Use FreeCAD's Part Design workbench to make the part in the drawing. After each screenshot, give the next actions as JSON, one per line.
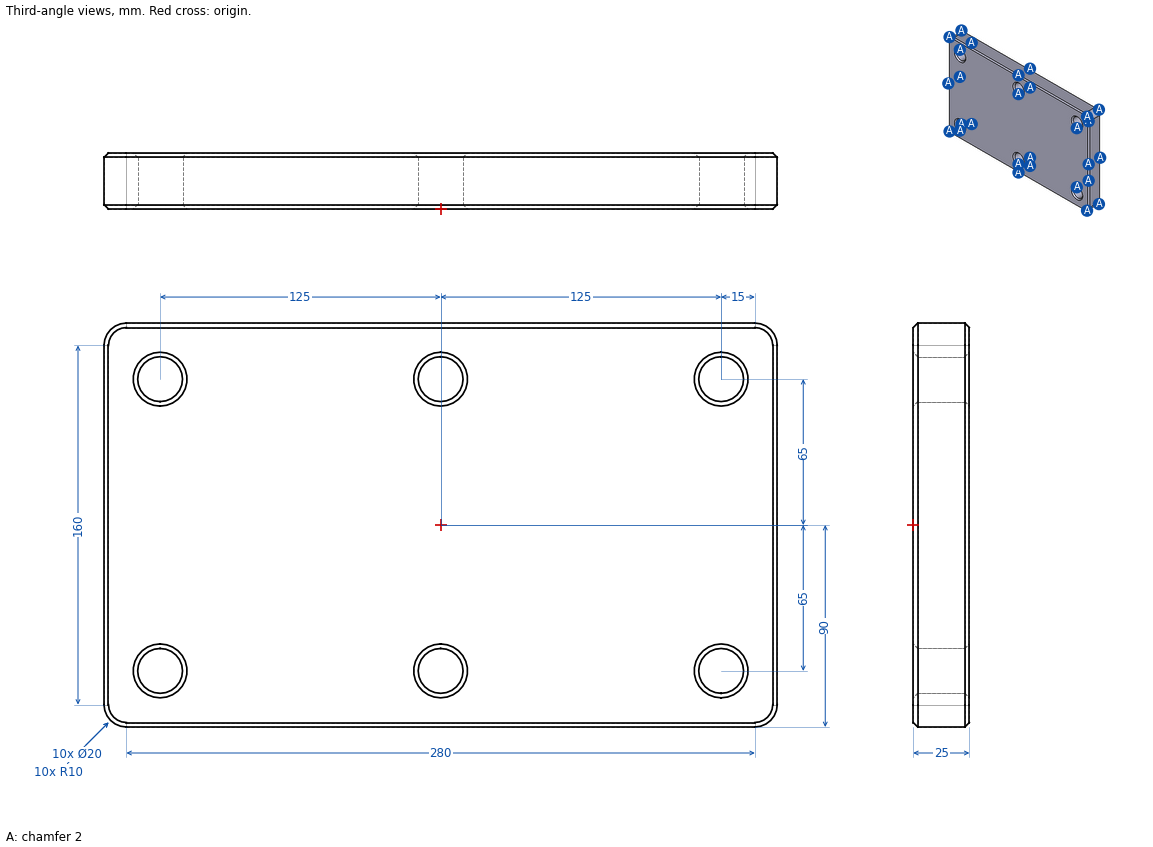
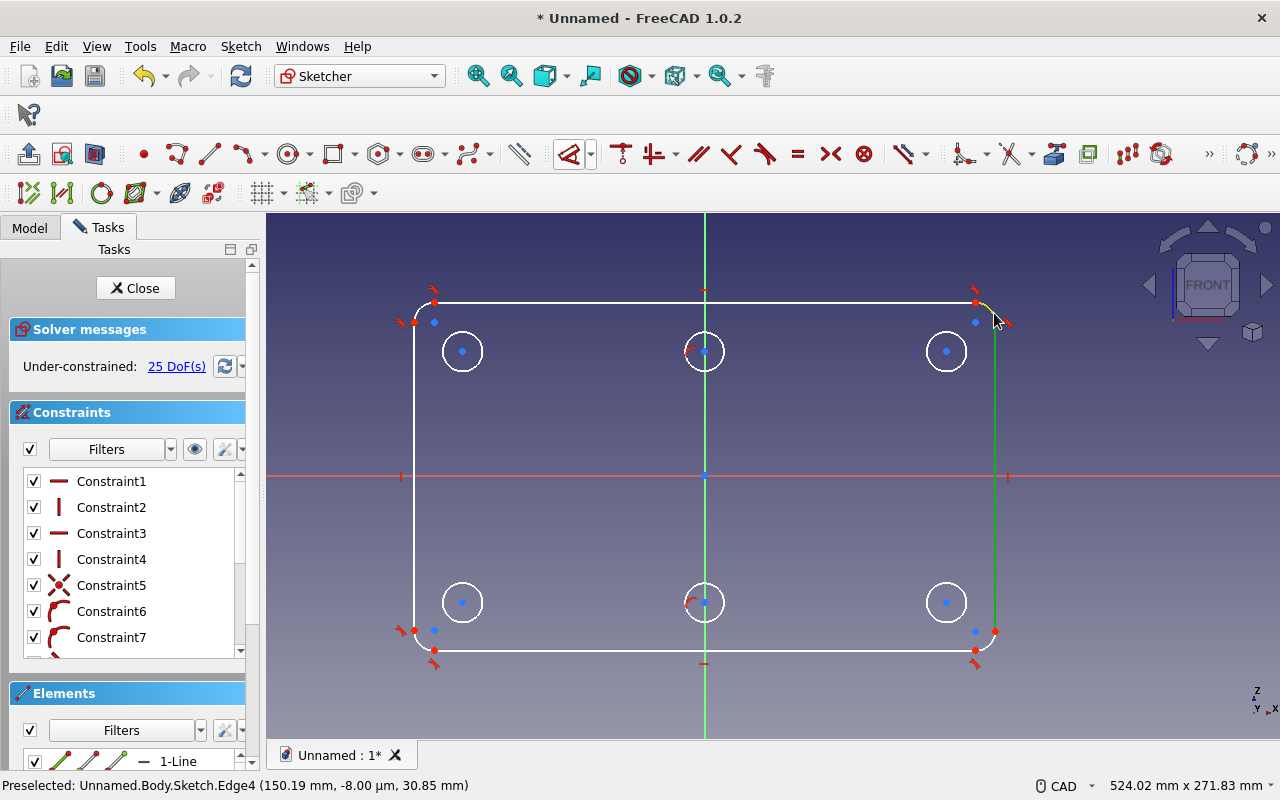
{"action": "scroll", "coordinate": [984, 649], "scroll_direction": "up", "scroll_amount": 3}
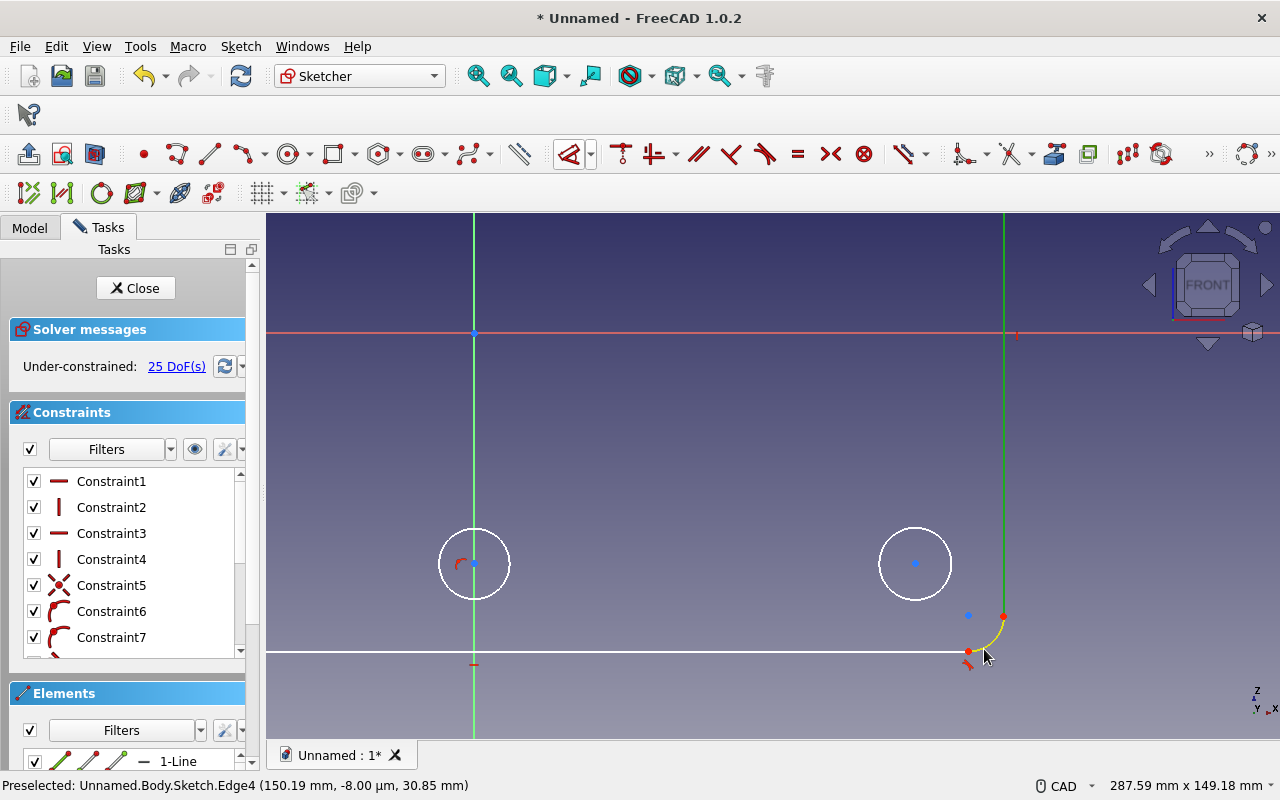
{"action": "left_click", "coordinate": [984, 648]}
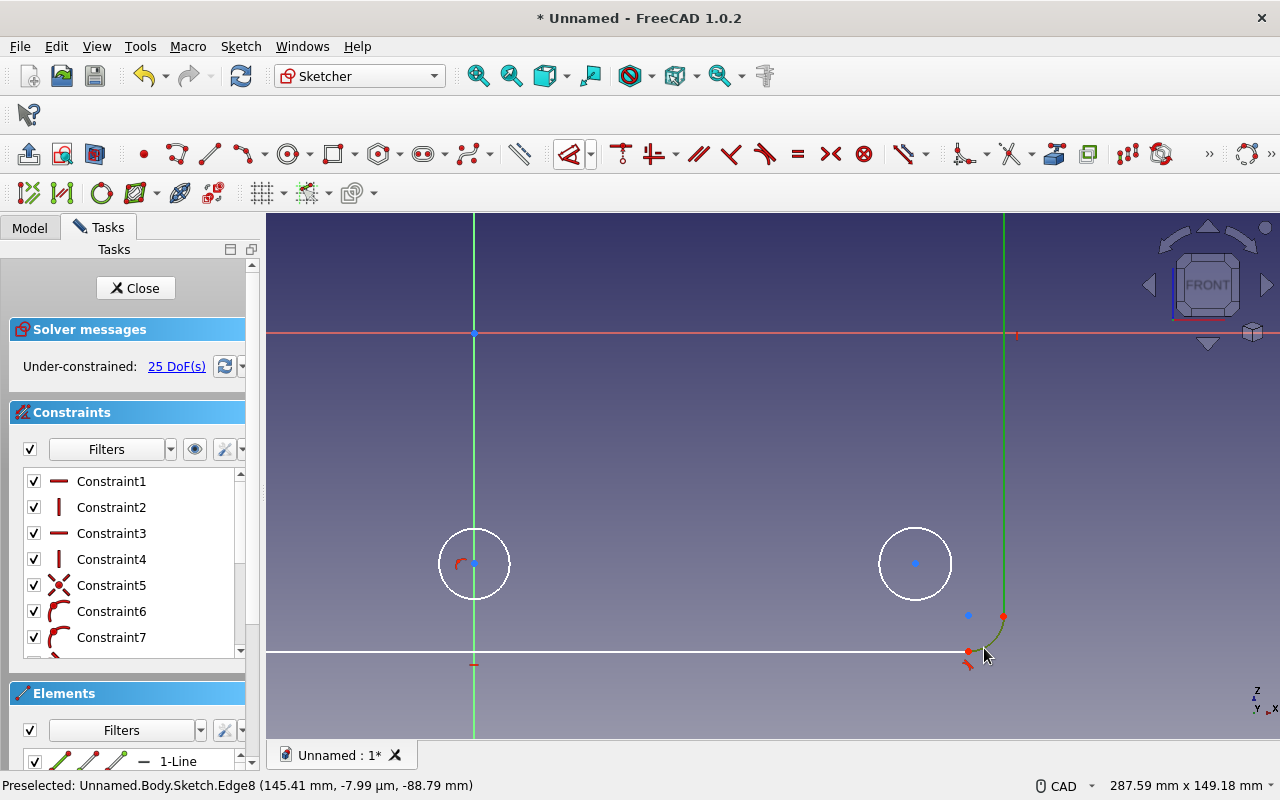
{"action": "left_click", "coordinate": [765, 154]}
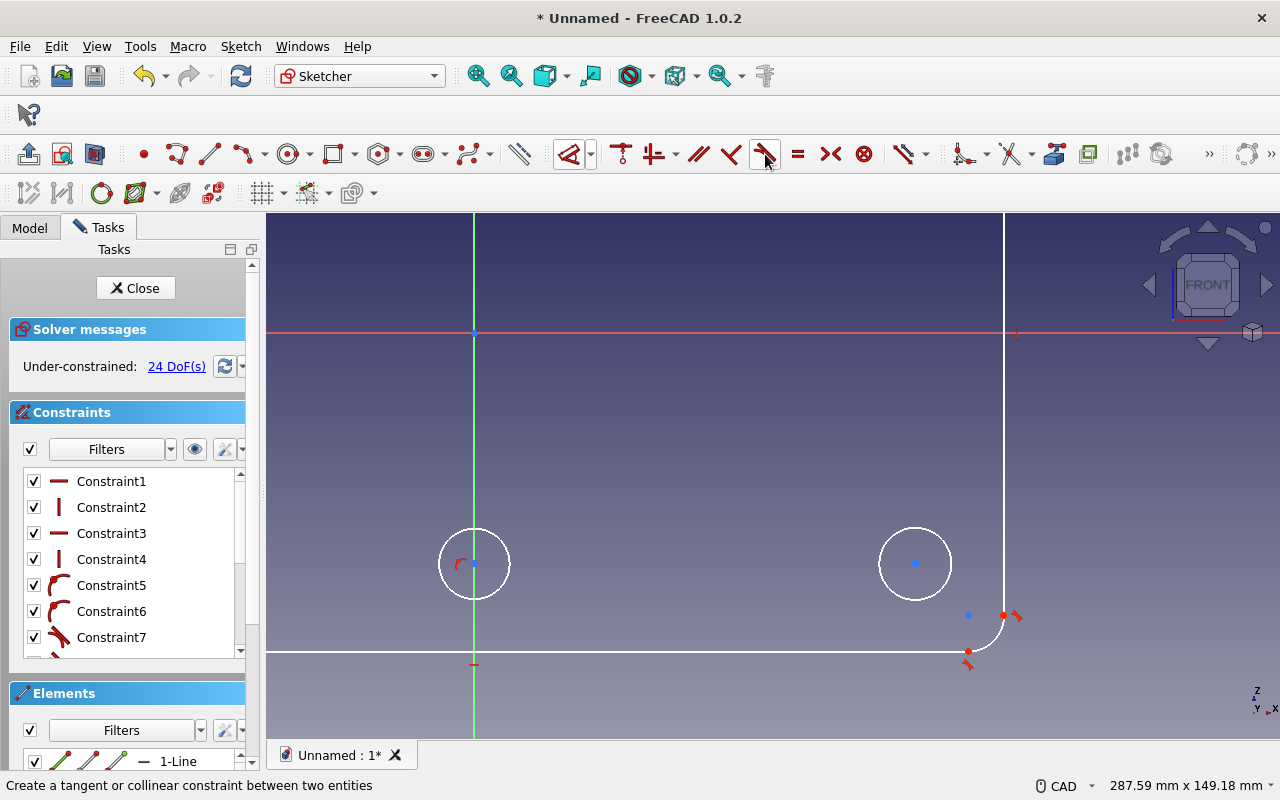
{"action": "scroll", "coordinate": [984, 650], "scroll_direction": "down", "scroll_amount": 3}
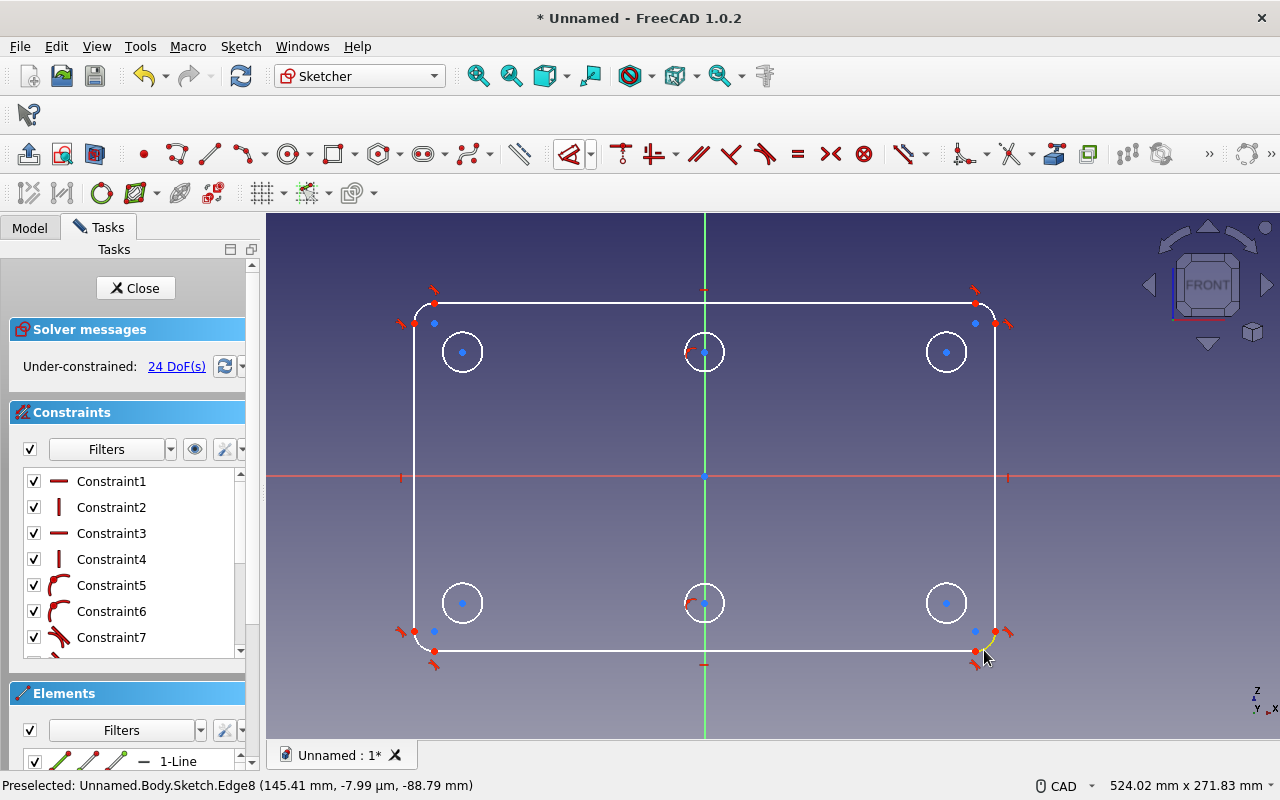
{"action": "scroll", "coordinate": [416, 640], "scroll_direction": "up", "scroll_amount": 3}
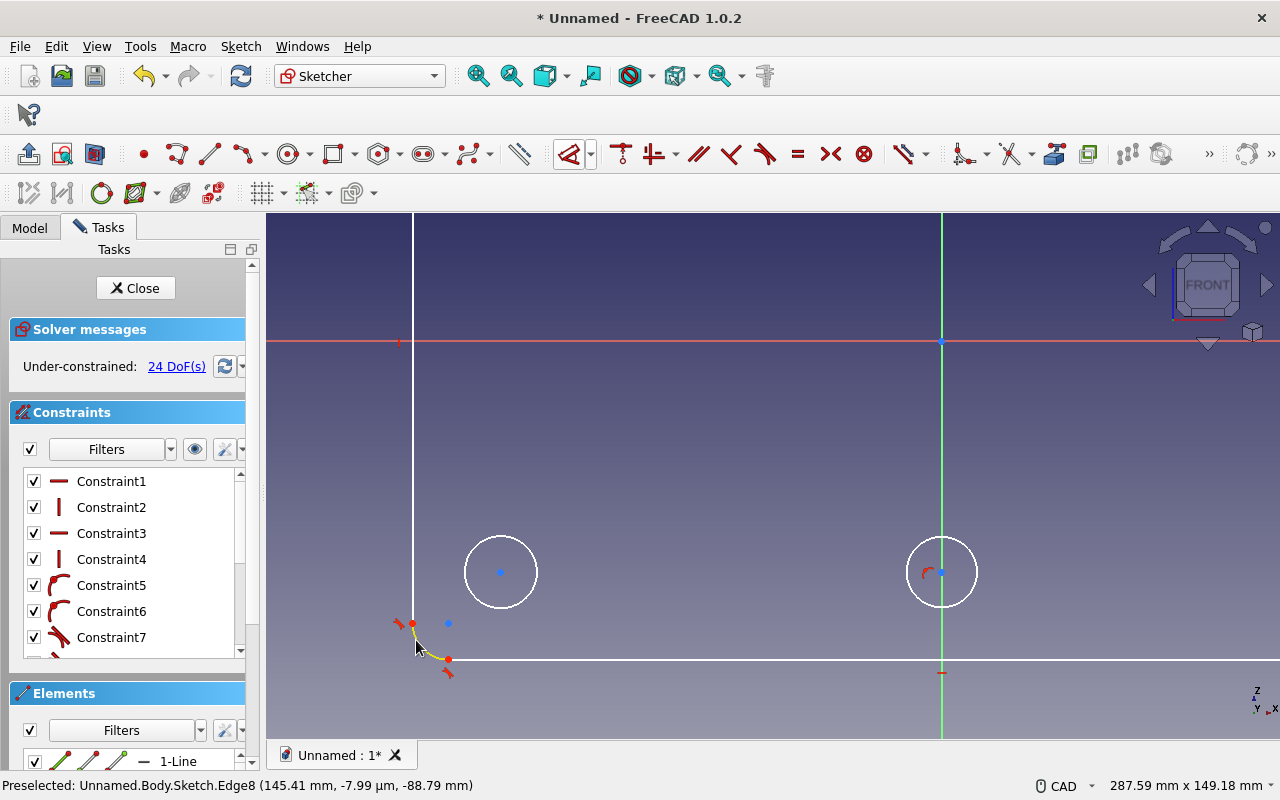
{"action": "left_click", "coordinate": [417, 640]}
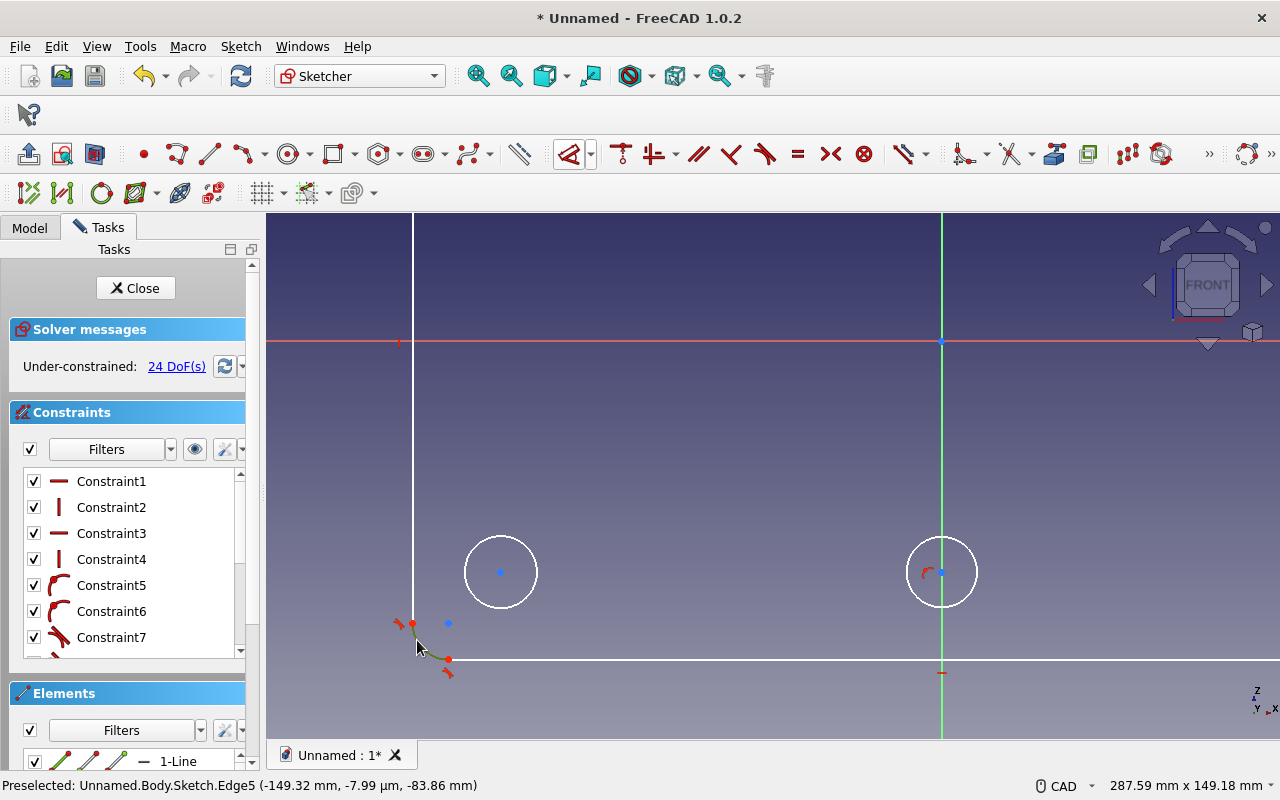
{"action": "scroll", "coordinate": [416, 640], "scroll_direction": "down", "scroll_amount": 3}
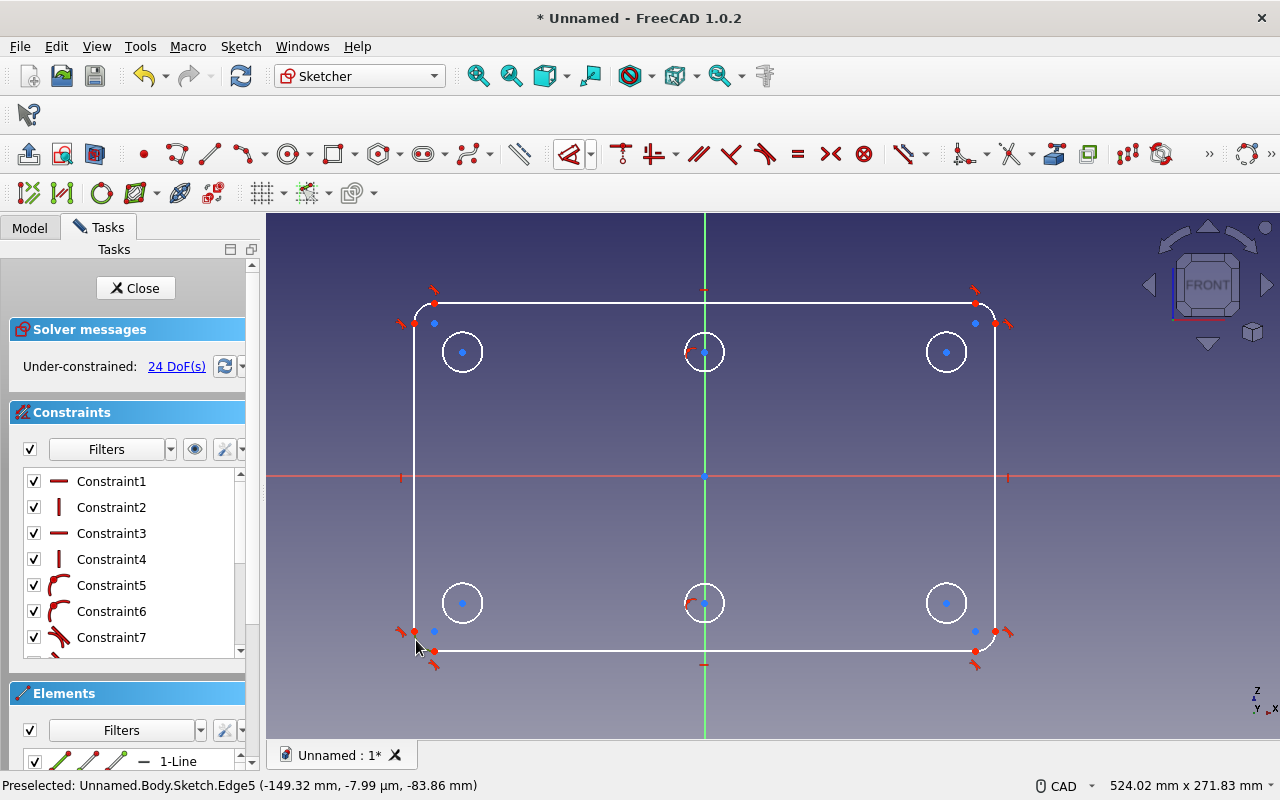
{"action": "scroll", "coordinate": [425, 305], "scroll_direction": "up", "scroll_amount": 2}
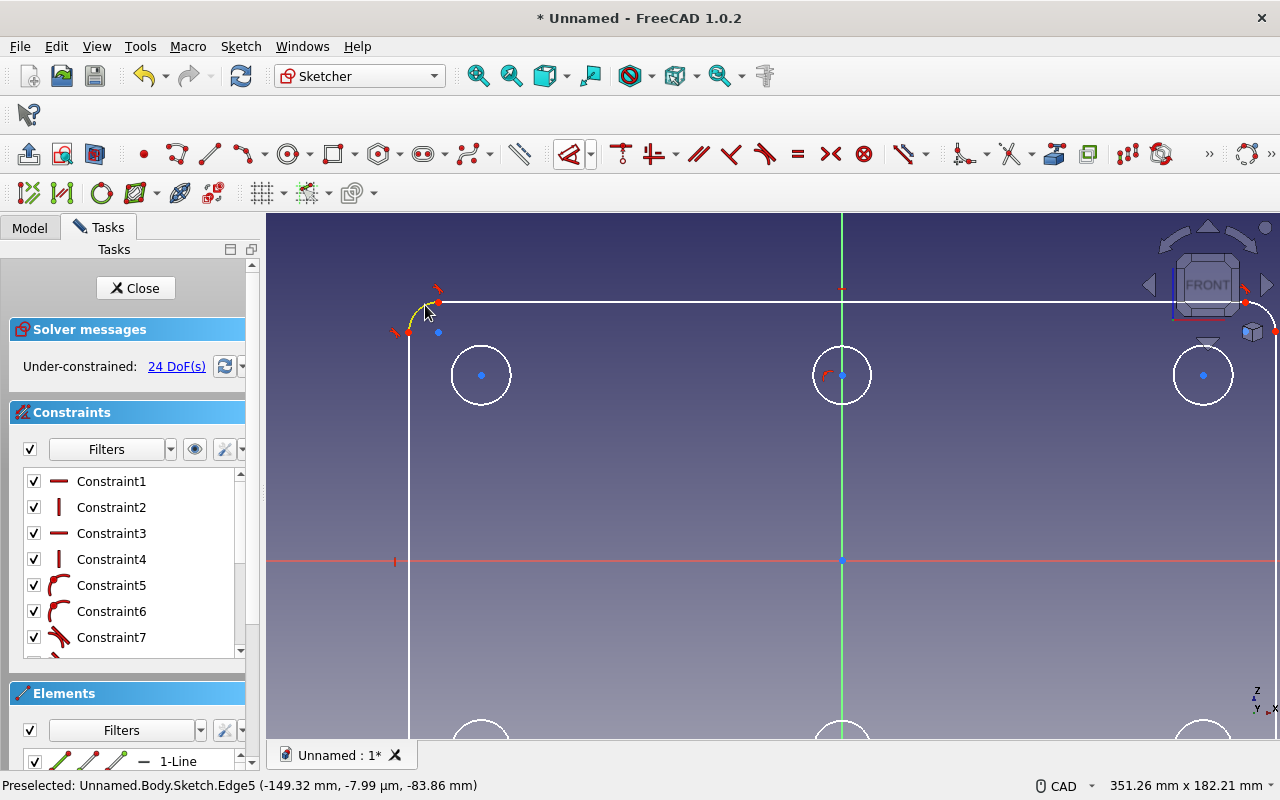
{"action": "left_click", "coordinate": [425, 305]}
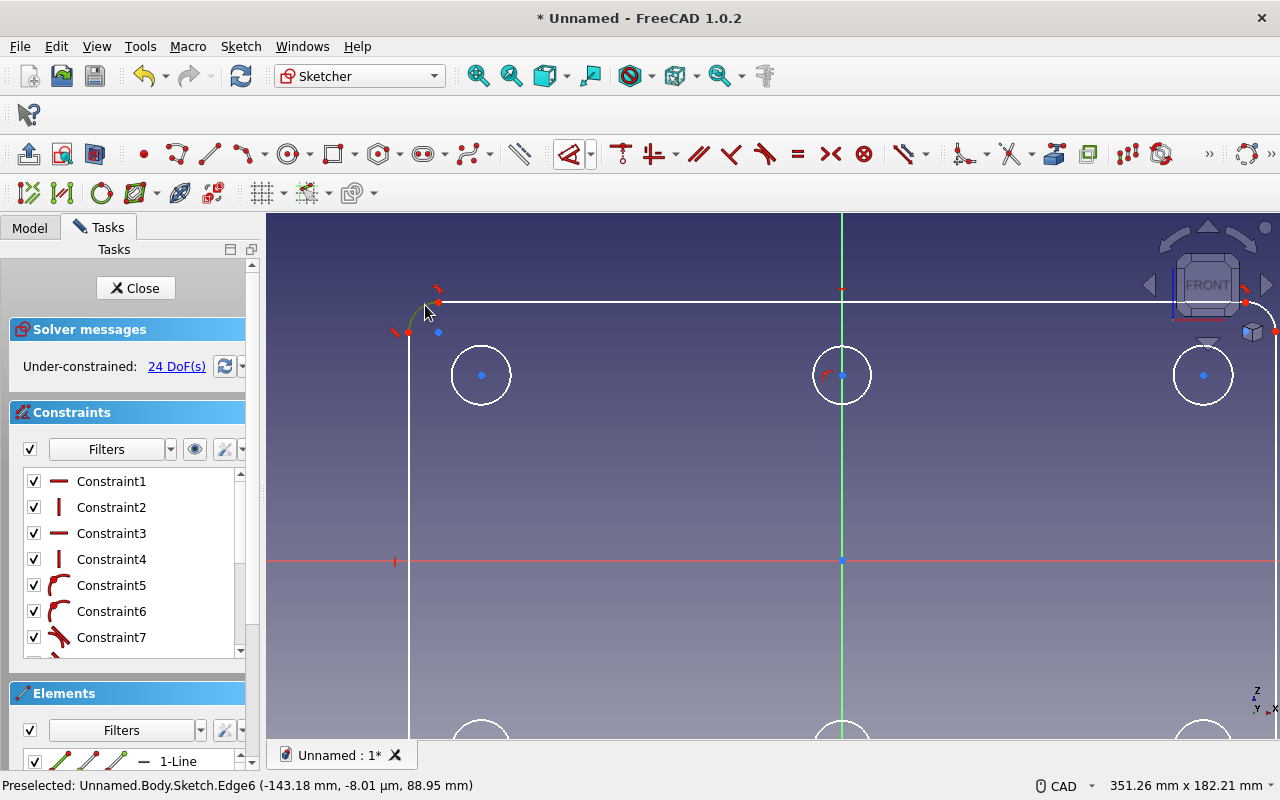
{"action": "scroll", "coordinate": [425, 304], "scroll_direction": "down", "scroll_amount": 2}